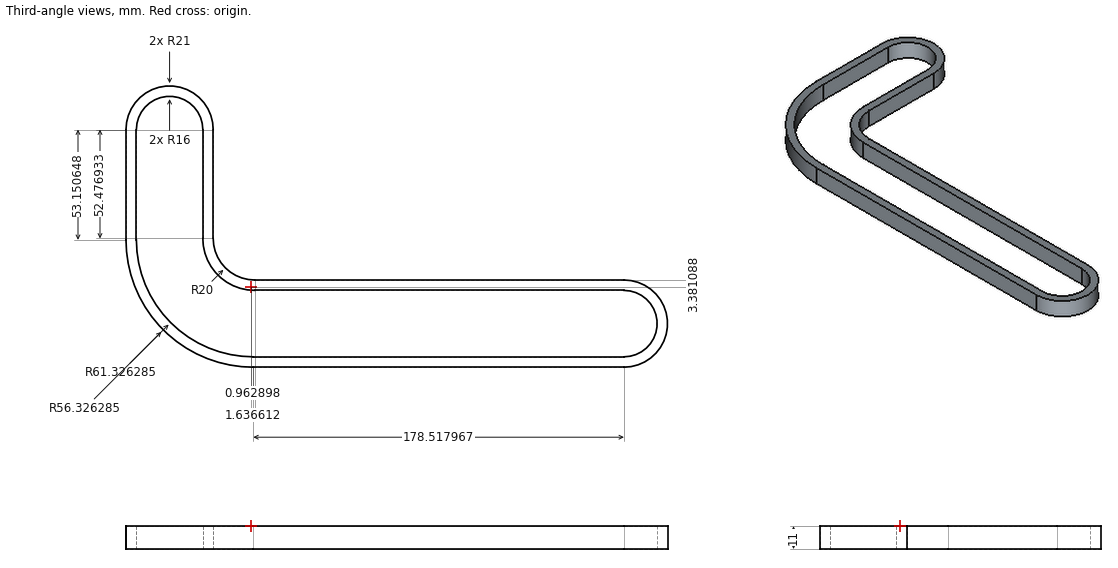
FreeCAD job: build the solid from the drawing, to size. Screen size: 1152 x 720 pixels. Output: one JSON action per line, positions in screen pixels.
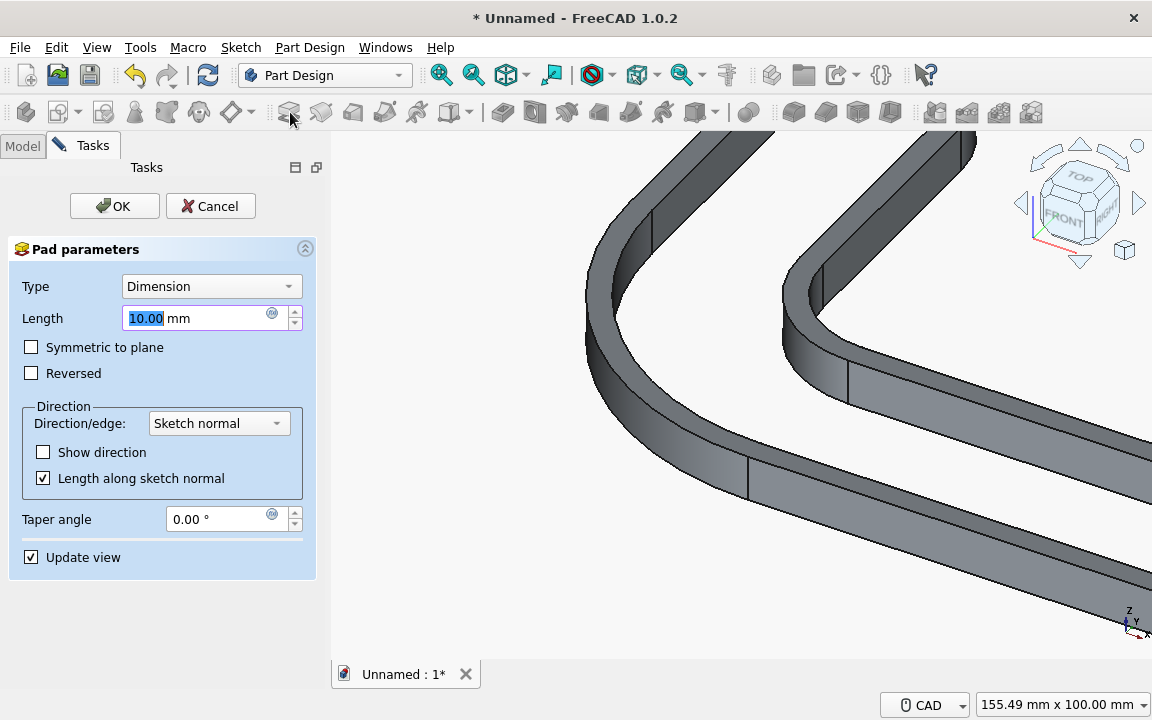
{"action": "type", "text": "11"}
{"action": "key", "text": "Tab"}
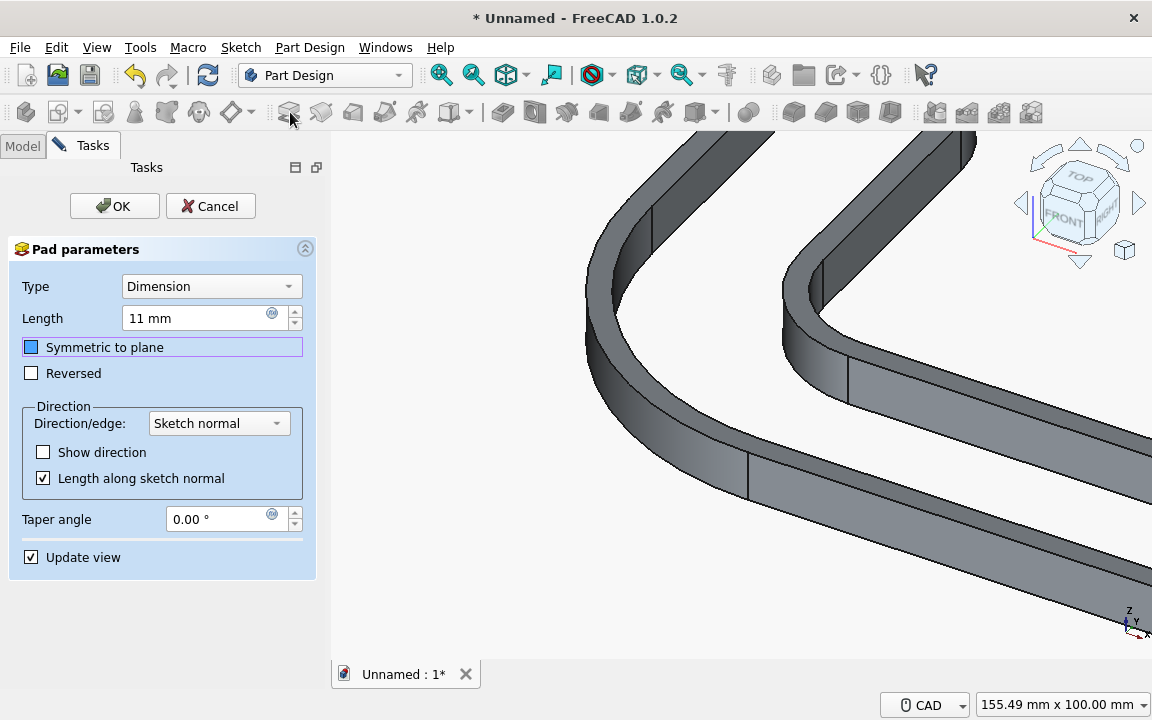
{"action": "left_click", "coordinate": [30, 373]}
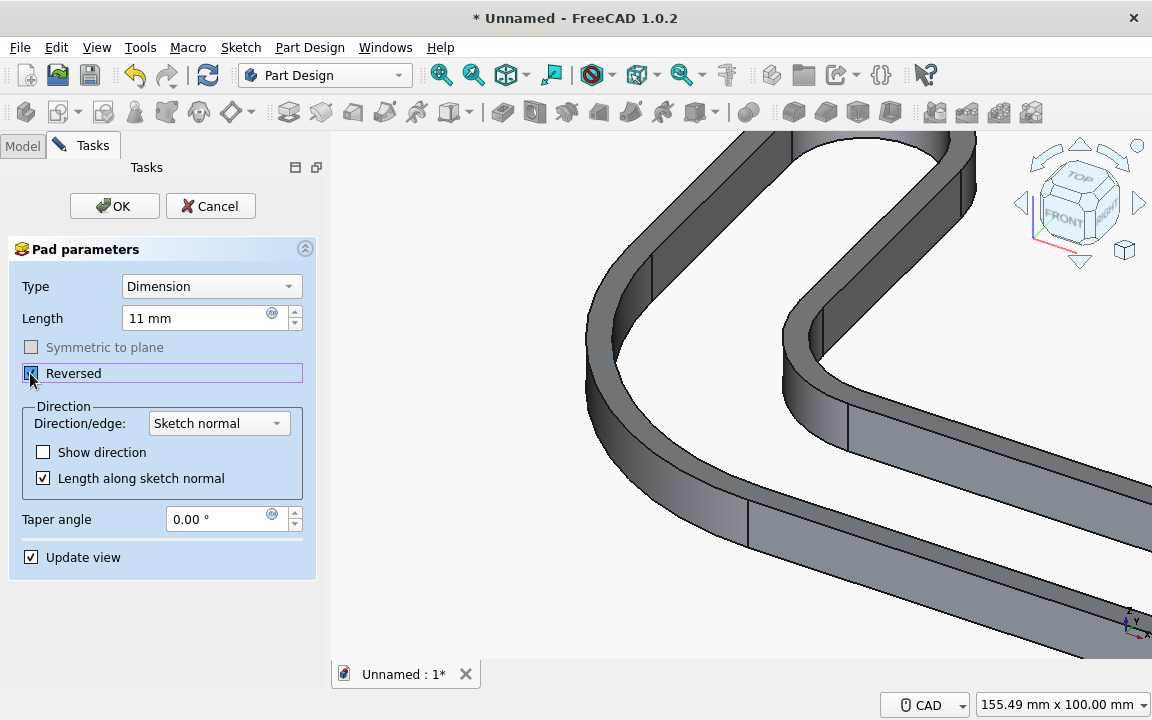
{"action": "left_click", "coordinate": [115, 206]}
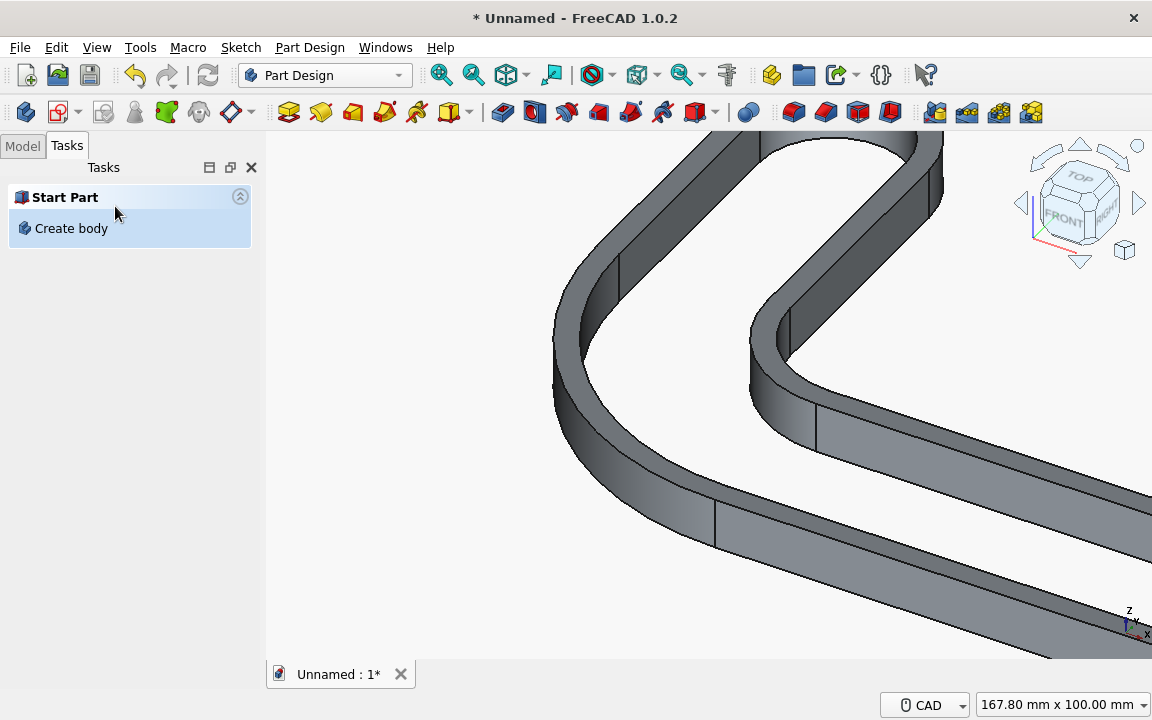
{"action": "key", "text": "0"}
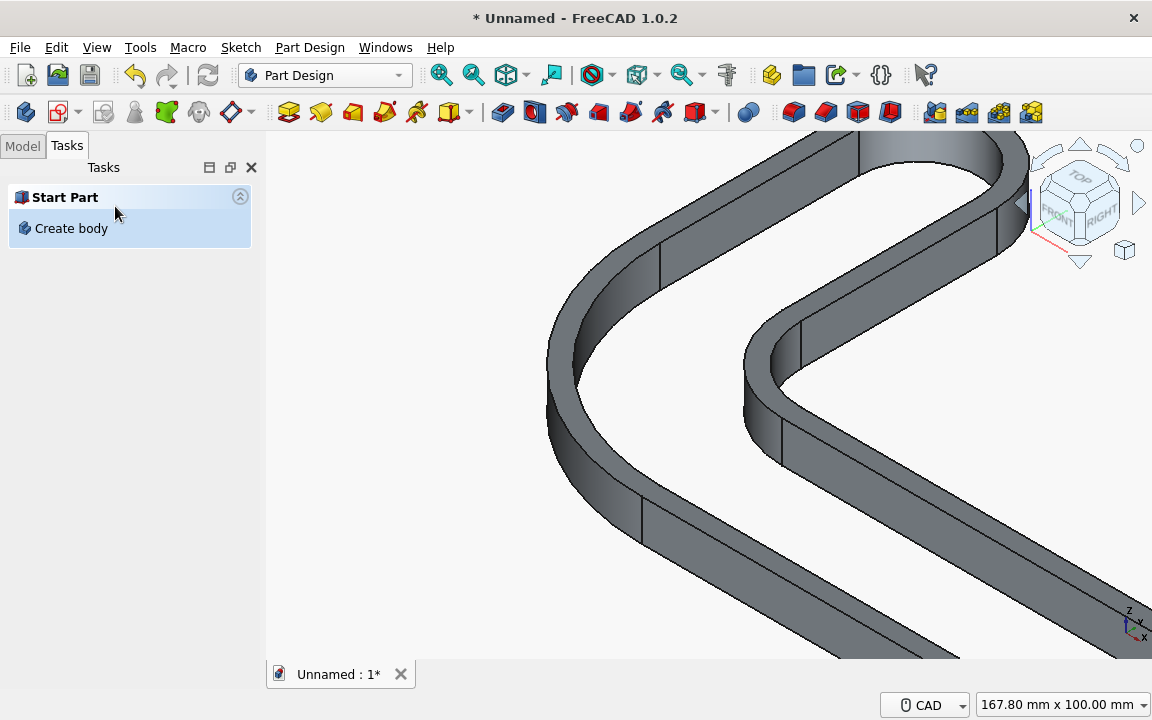
{"action": "left_click", "coordinate": [442, 76]}